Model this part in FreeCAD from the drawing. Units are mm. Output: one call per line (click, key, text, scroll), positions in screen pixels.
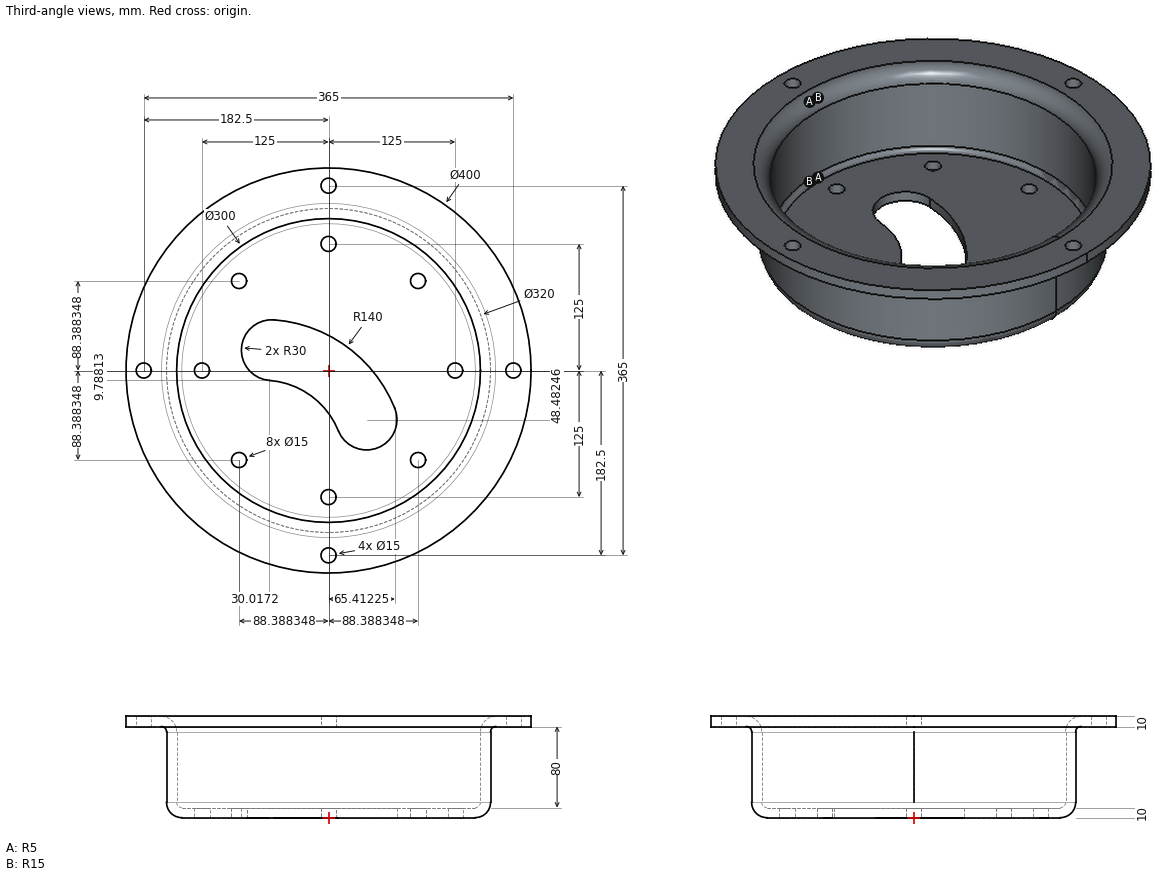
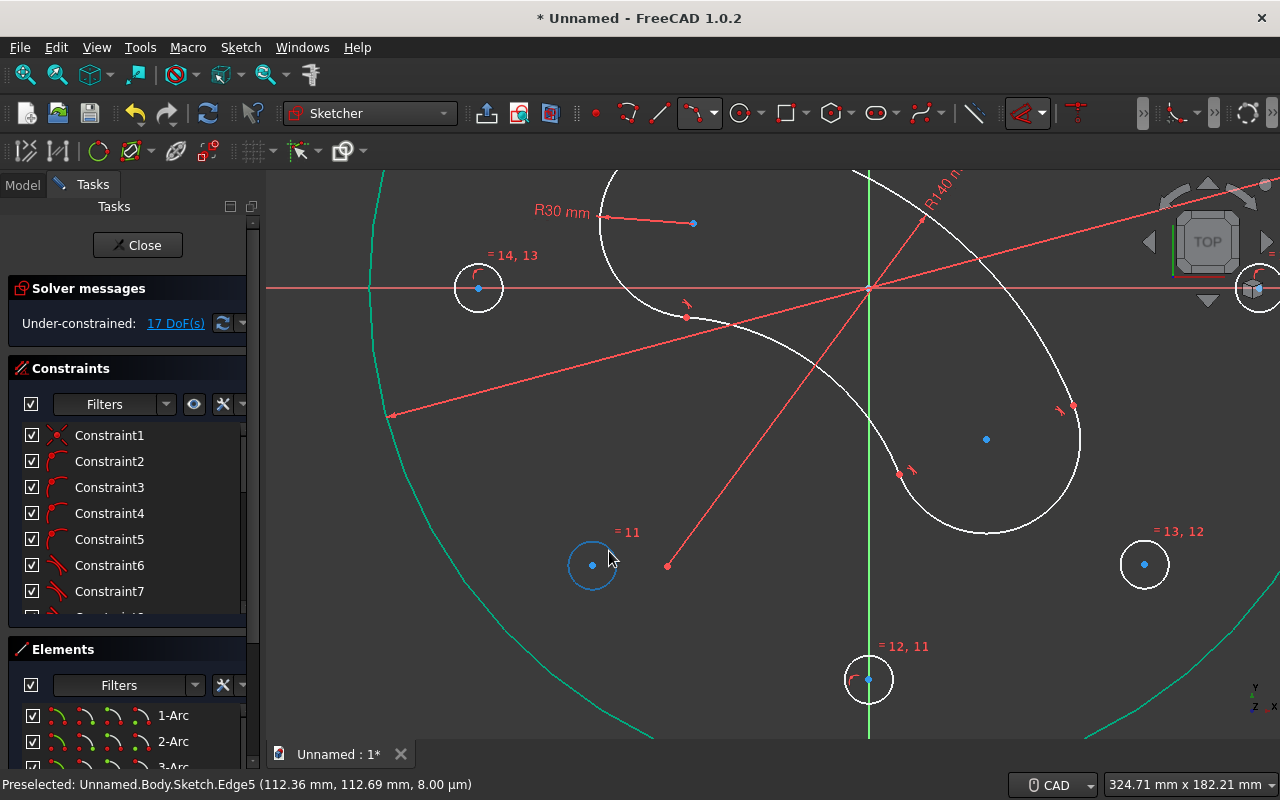
click(609, 549)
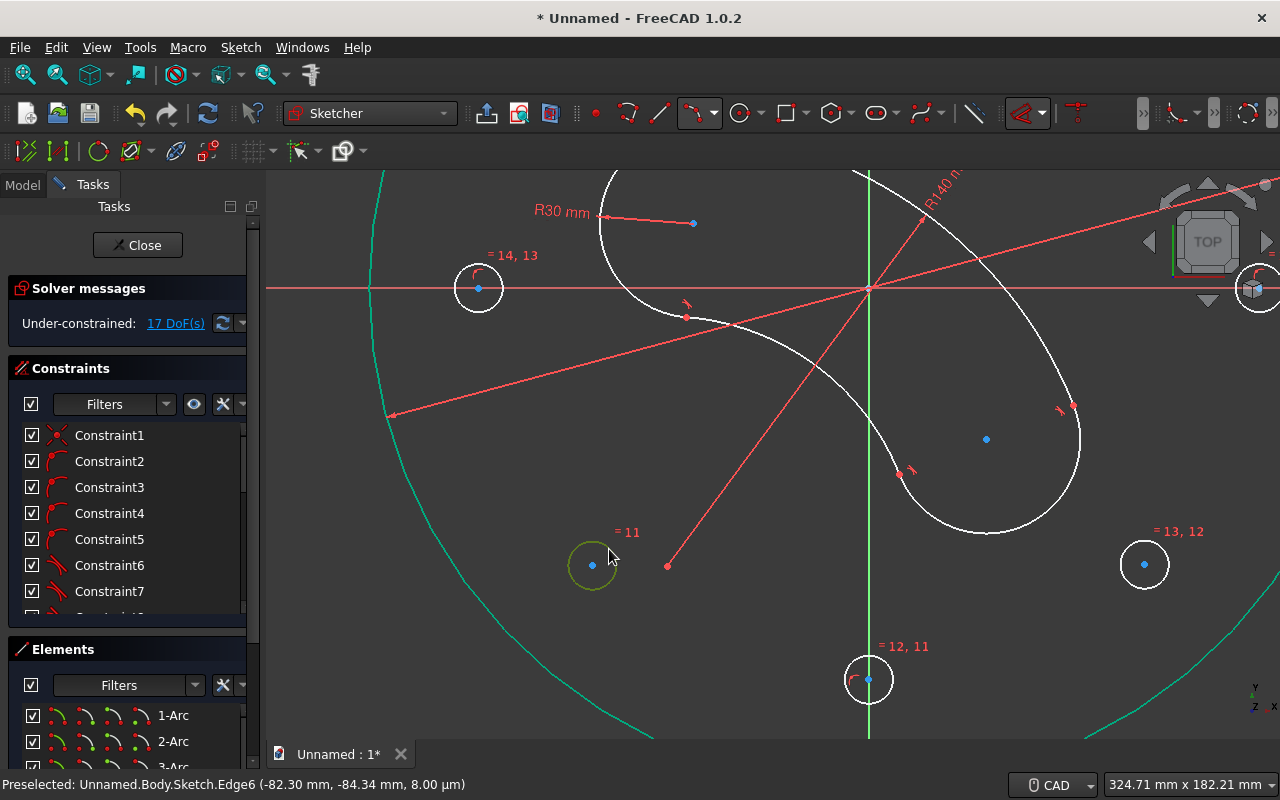
click(1044, 114)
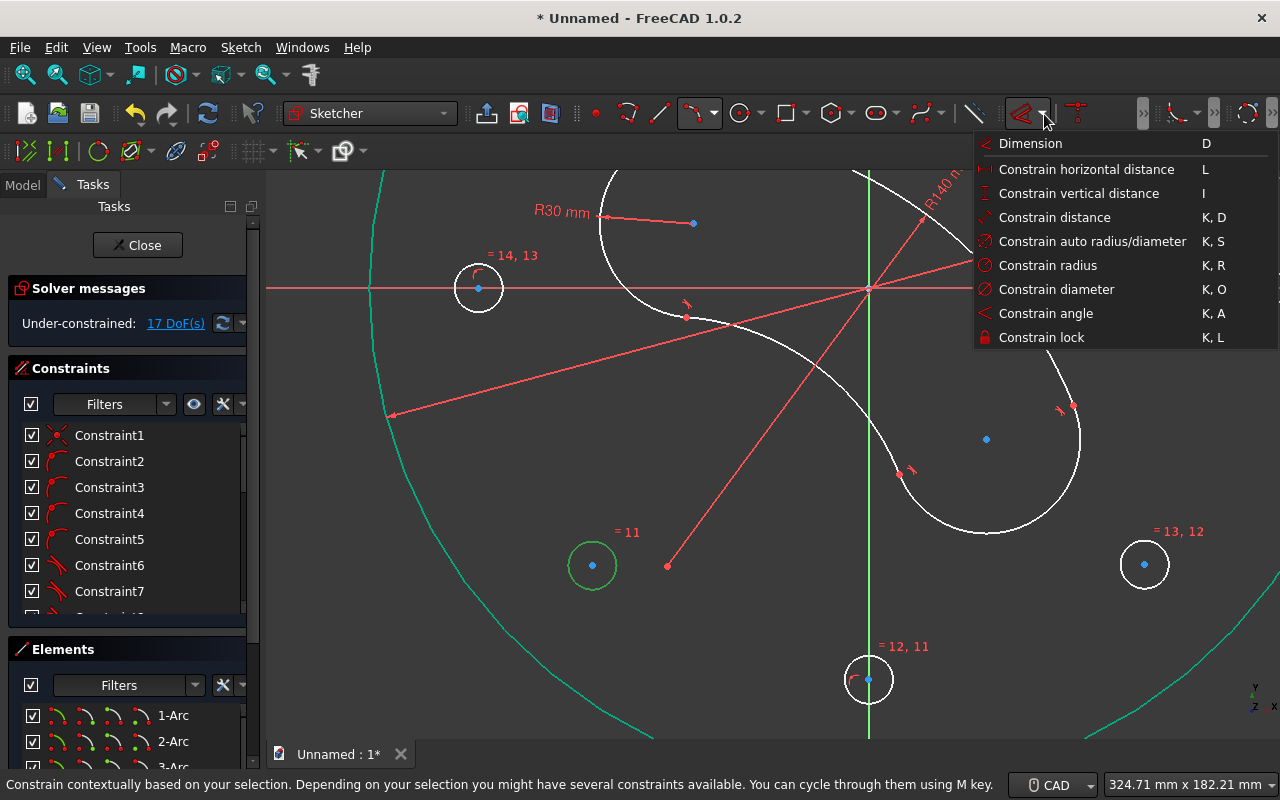
click(1126, 289)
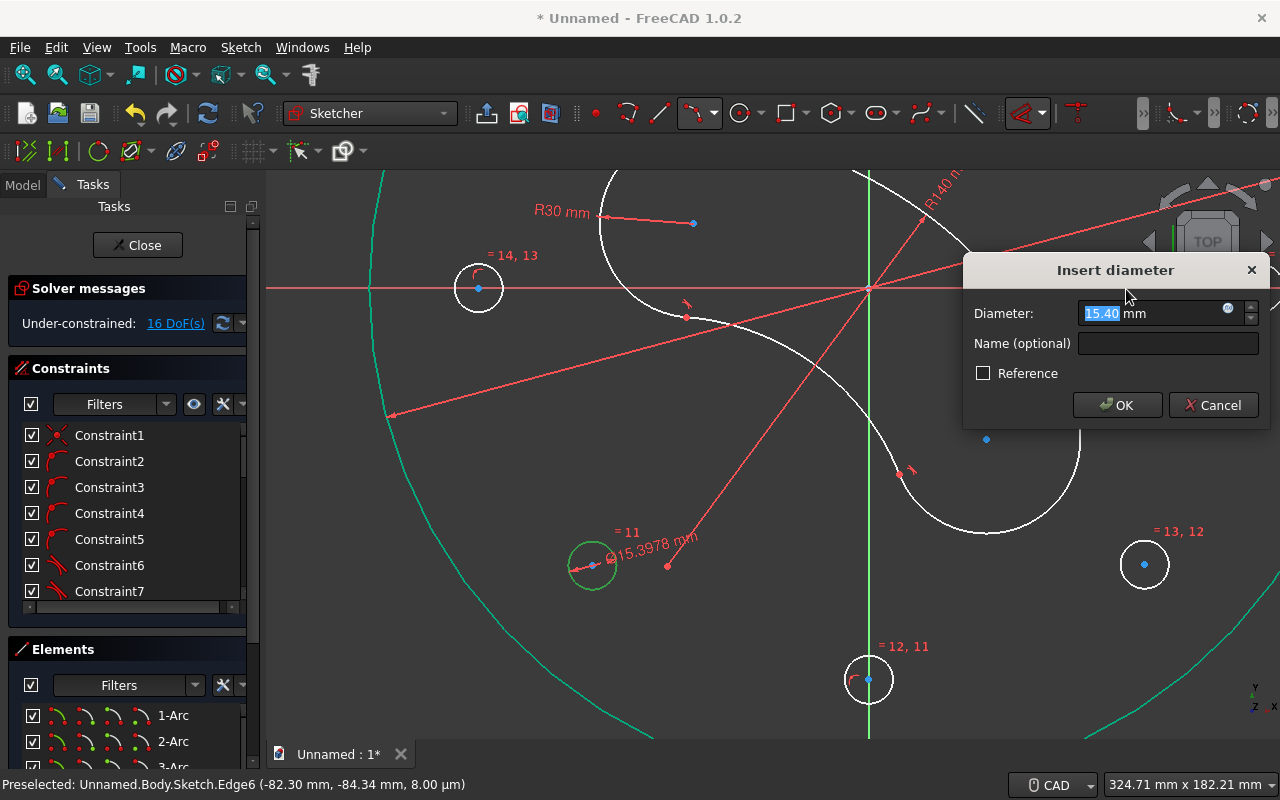
text(15)
key(Return)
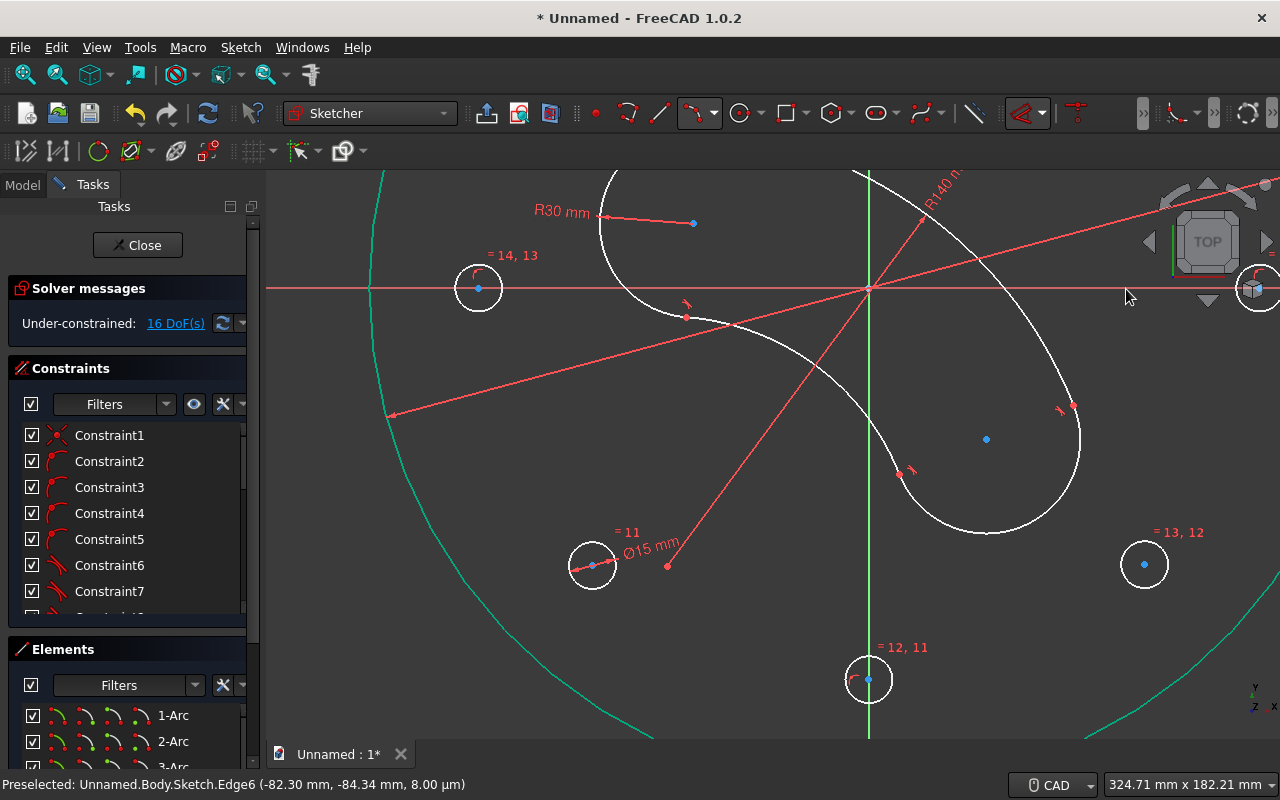
click(869, 680)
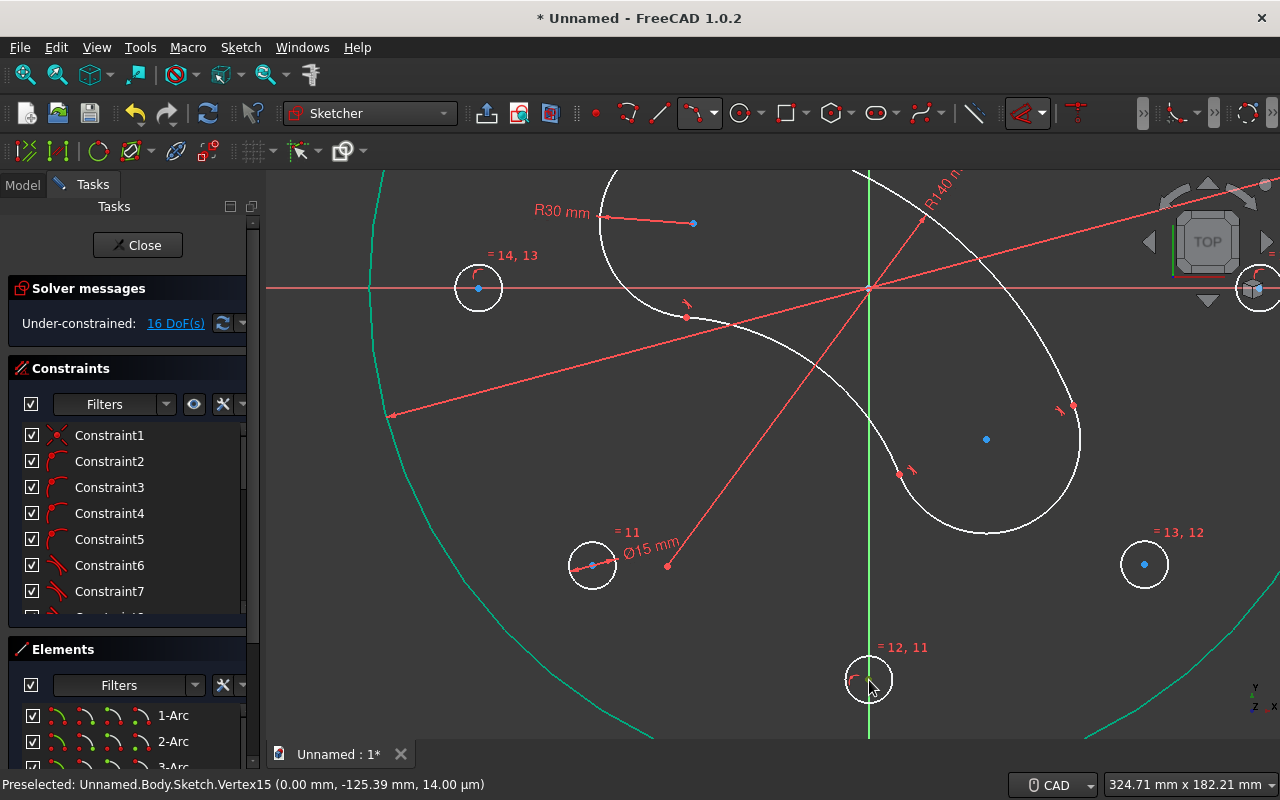
click(1044, 114)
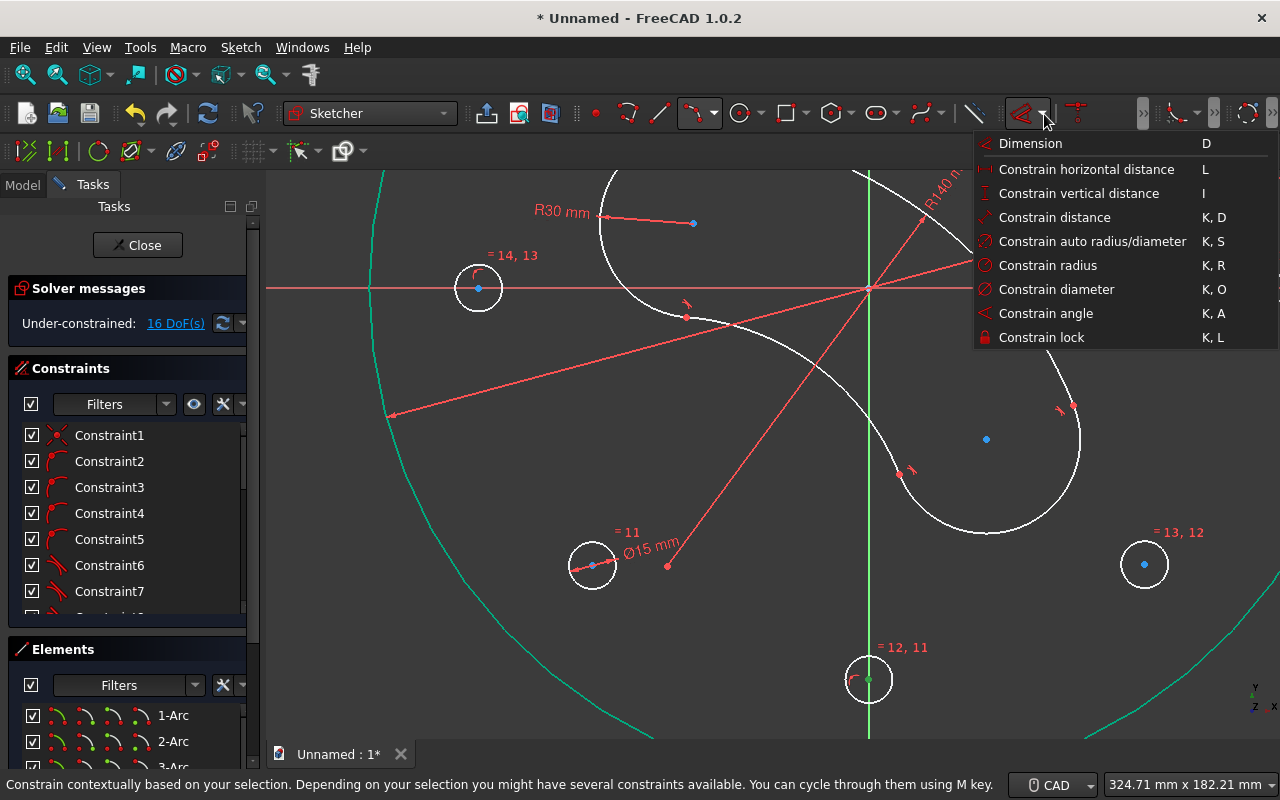
click(1126, 193)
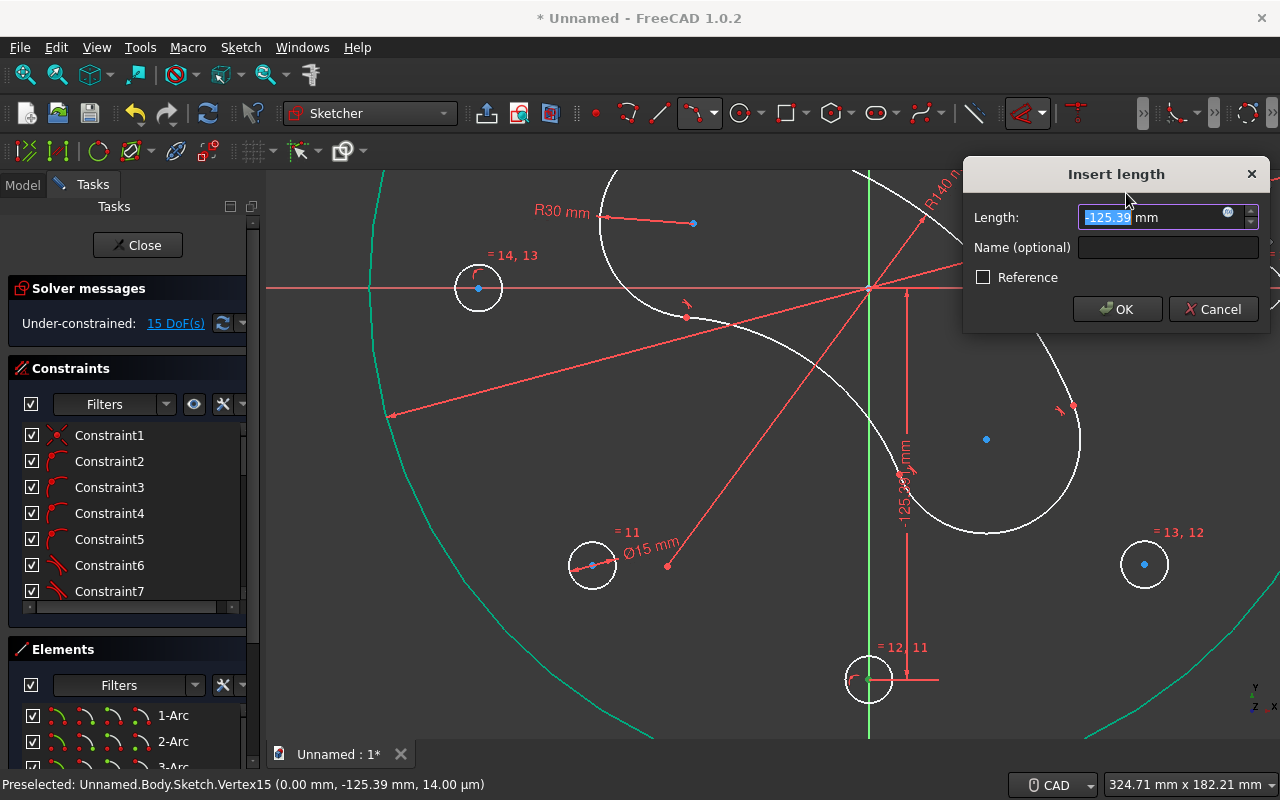
text(-125)
key(Return)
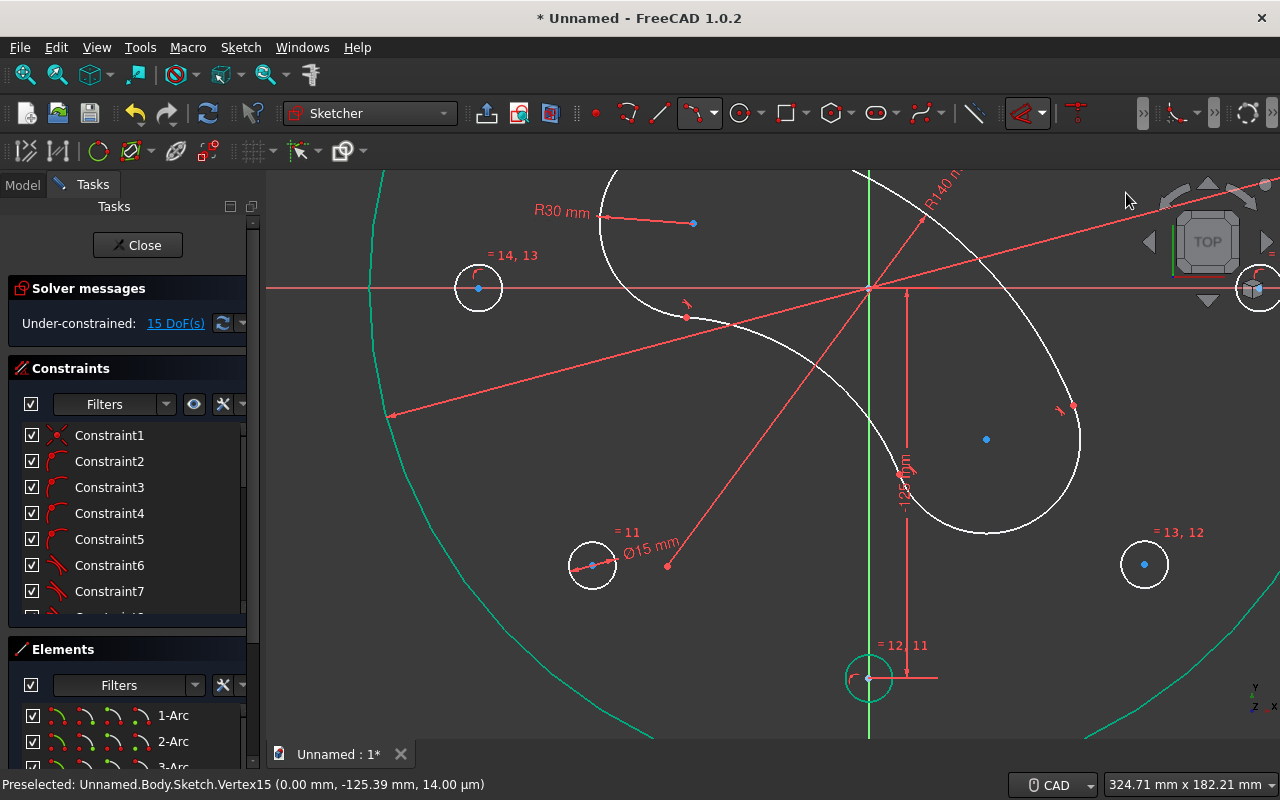
click(479, 288)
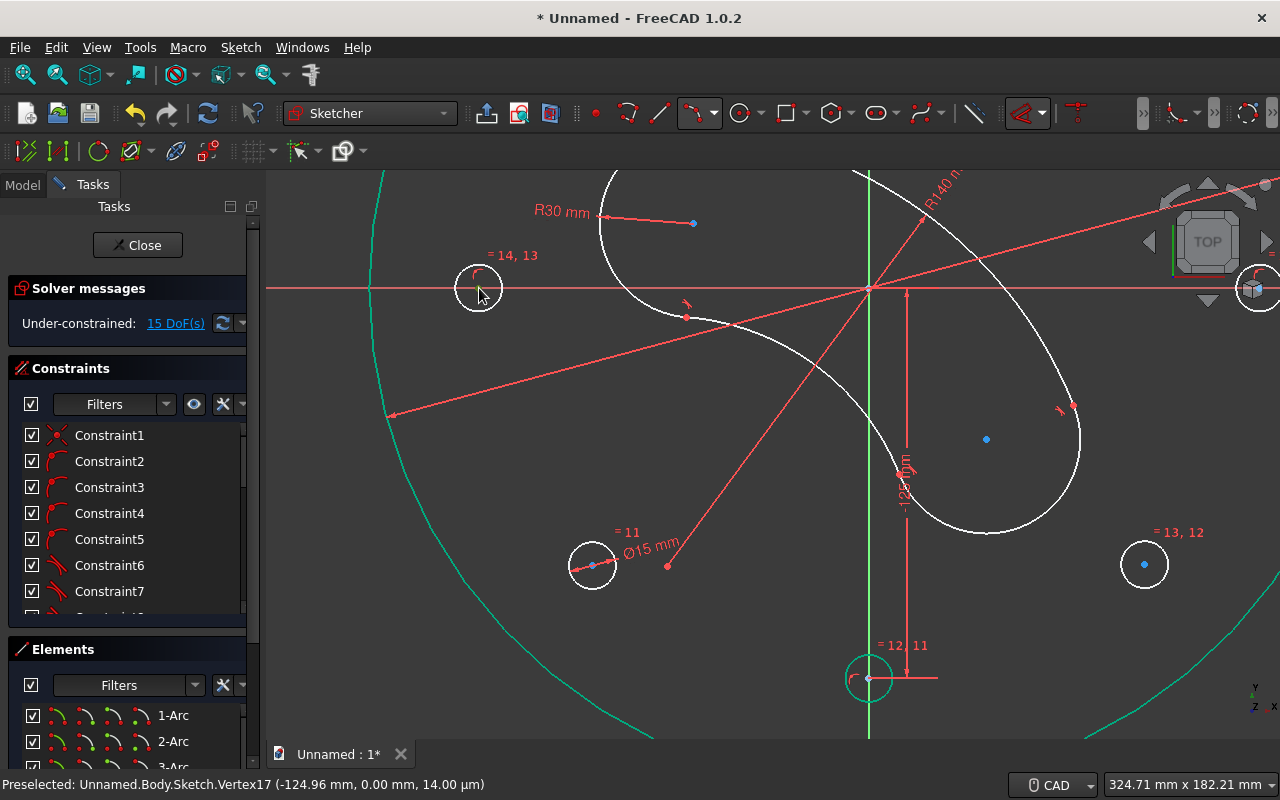
click(1044, 114)